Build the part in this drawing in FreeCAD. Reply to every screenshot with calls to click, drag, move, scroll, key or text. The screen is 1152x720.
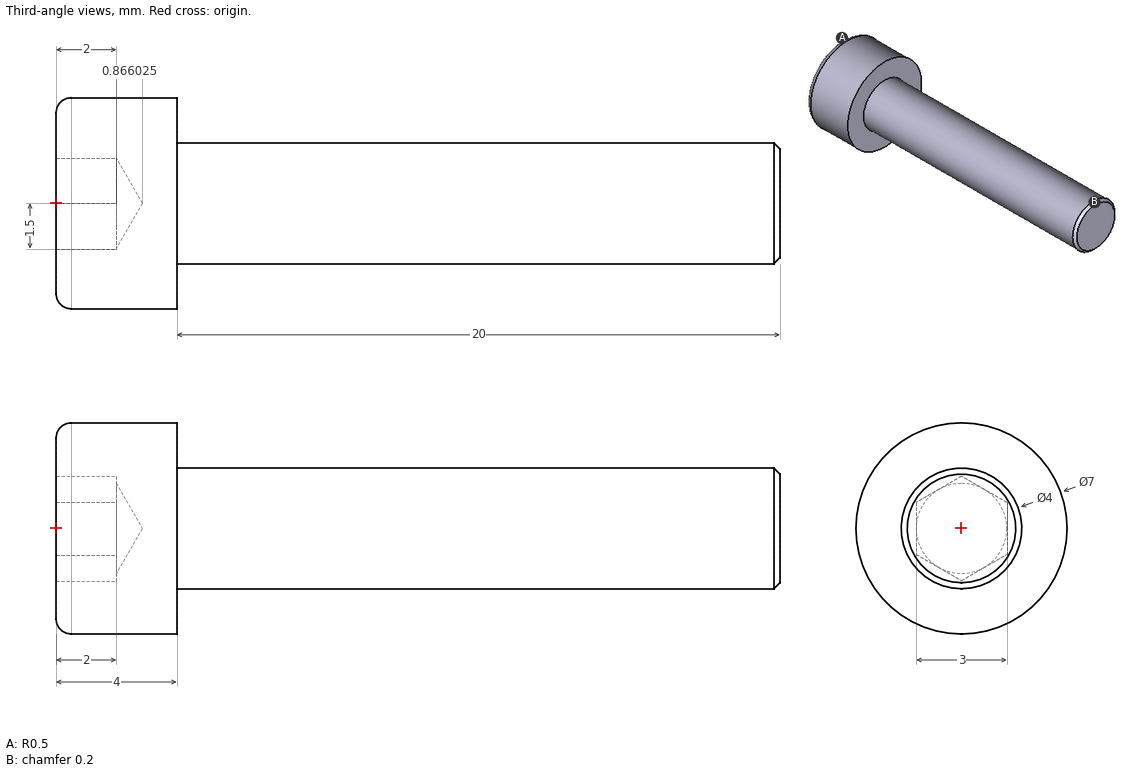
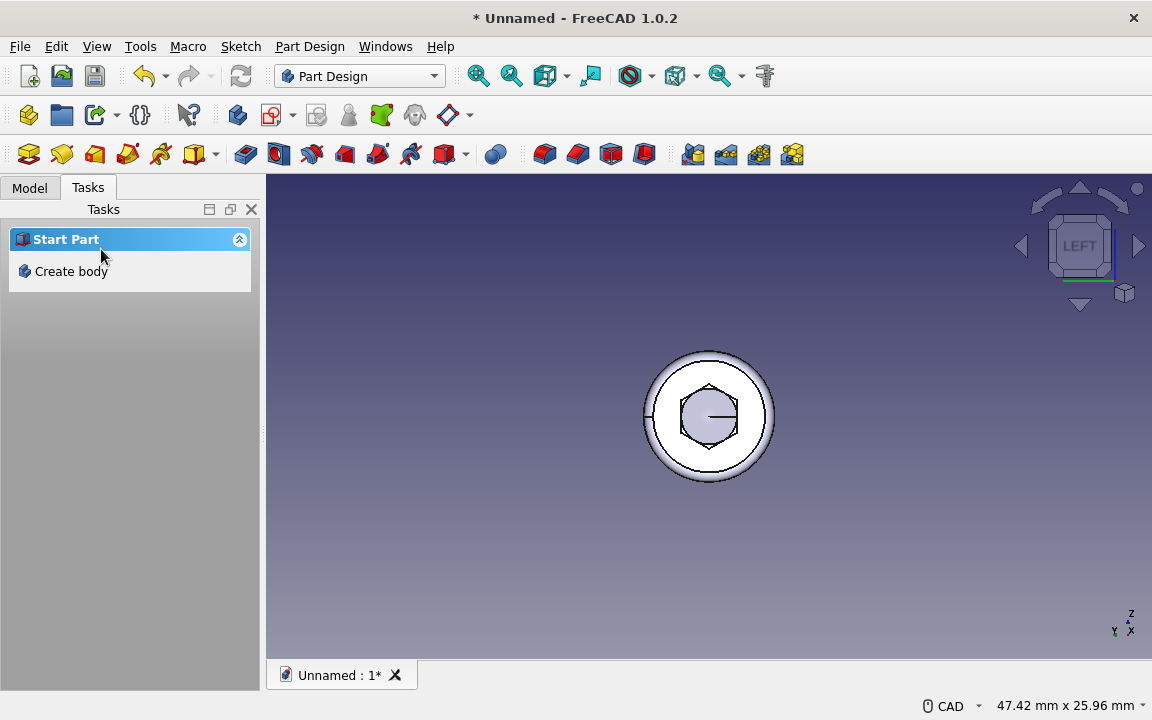
click(479, 76)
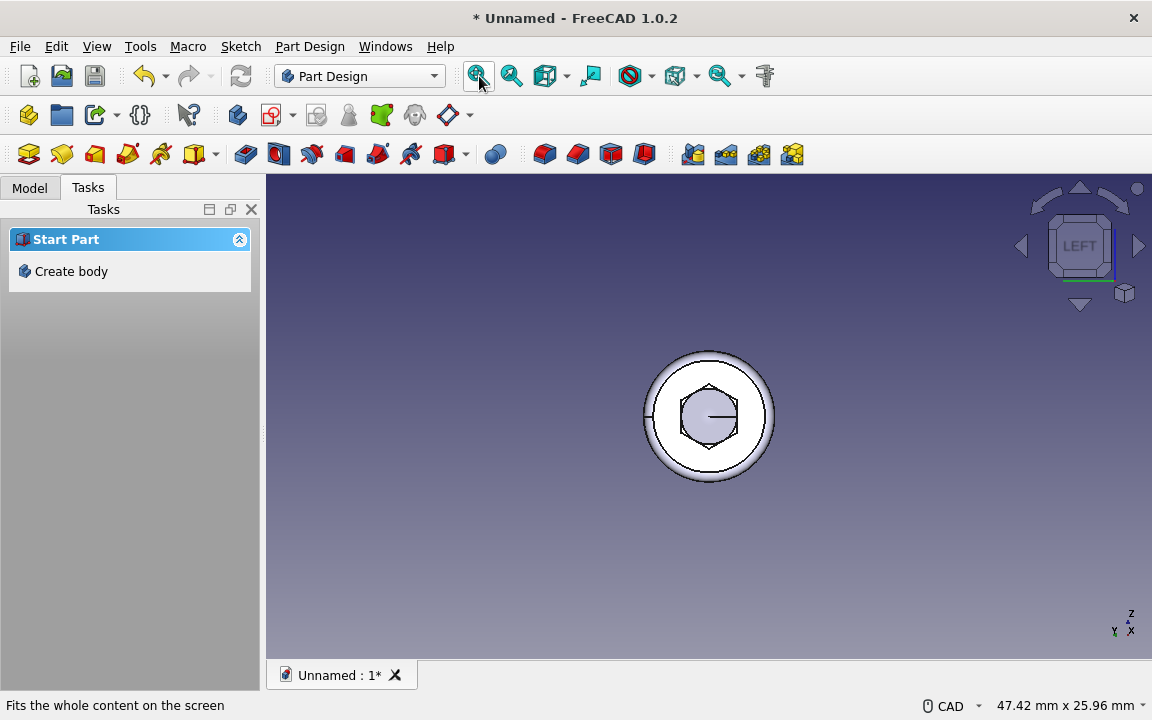
key(0)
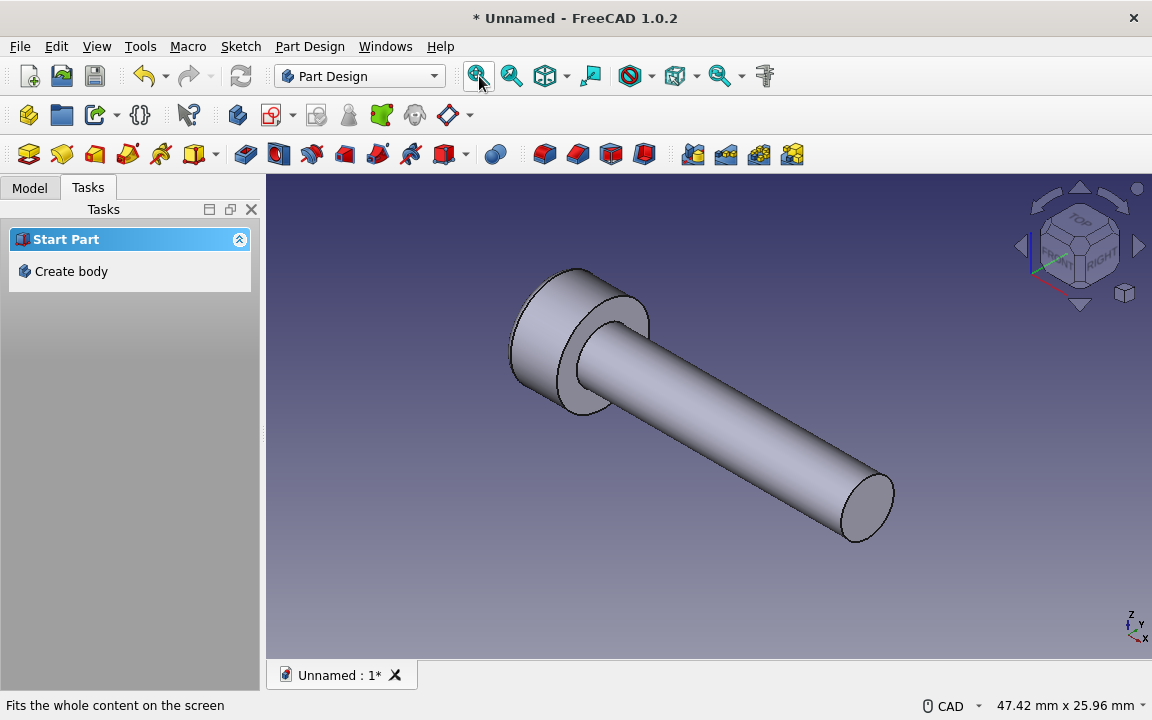
click(841, 522)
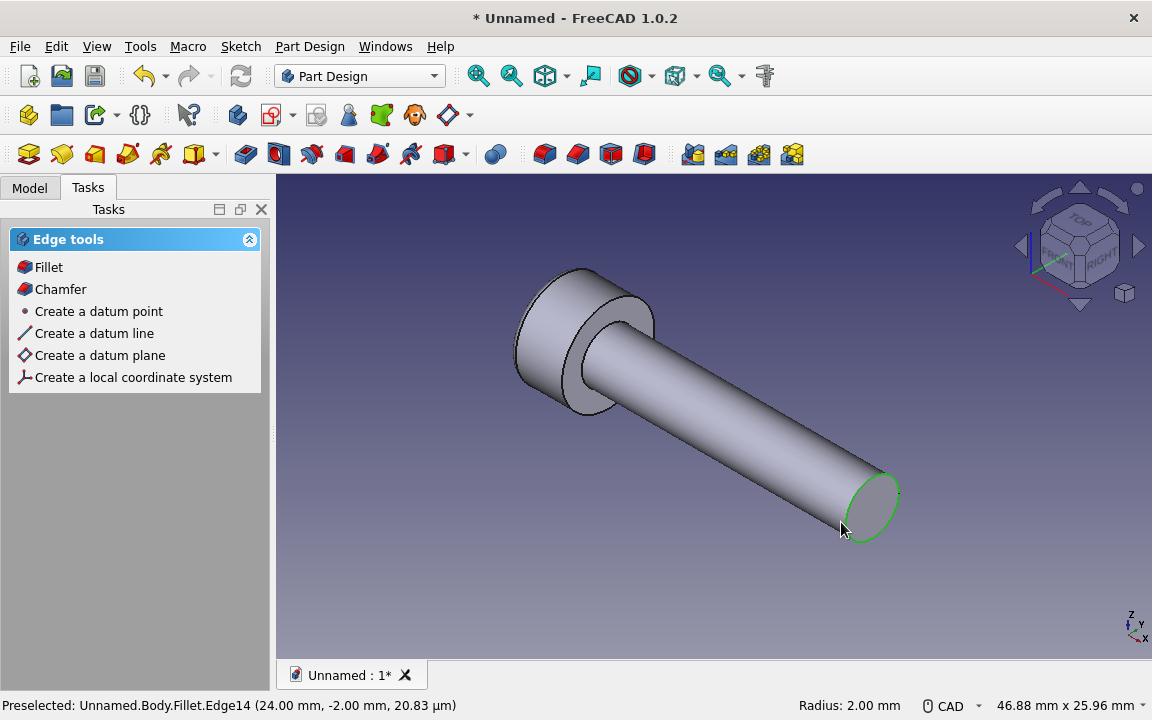
click(578, 154)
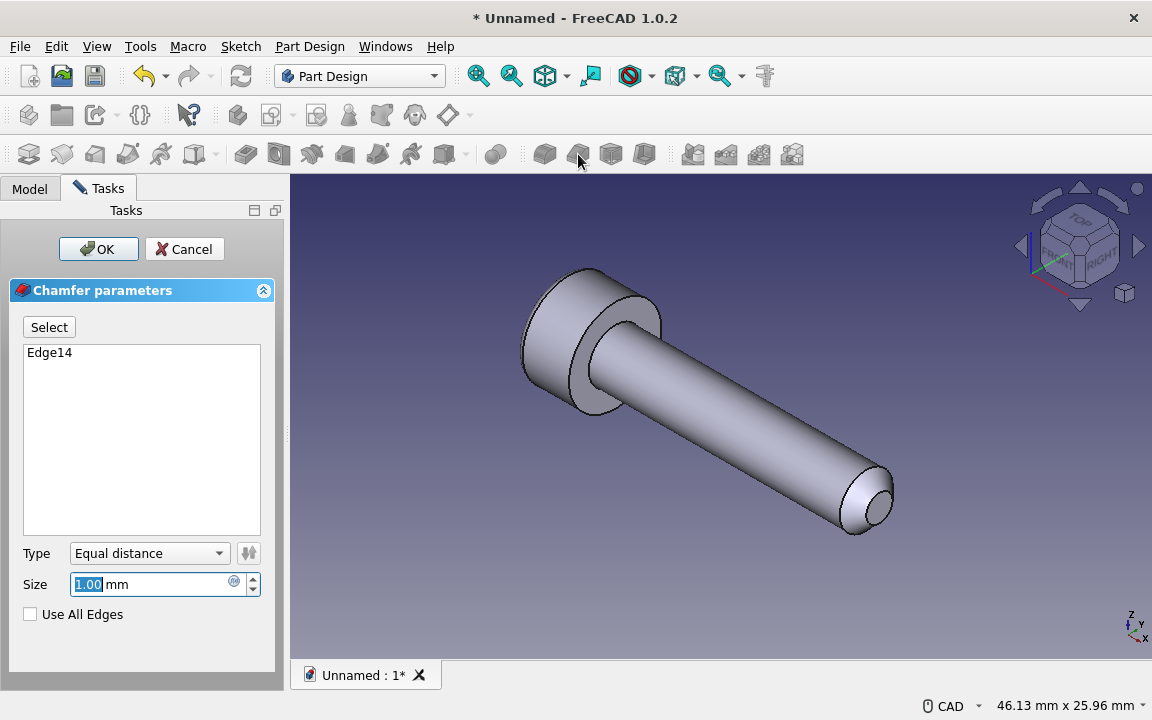
text(0.2)
key(Tab)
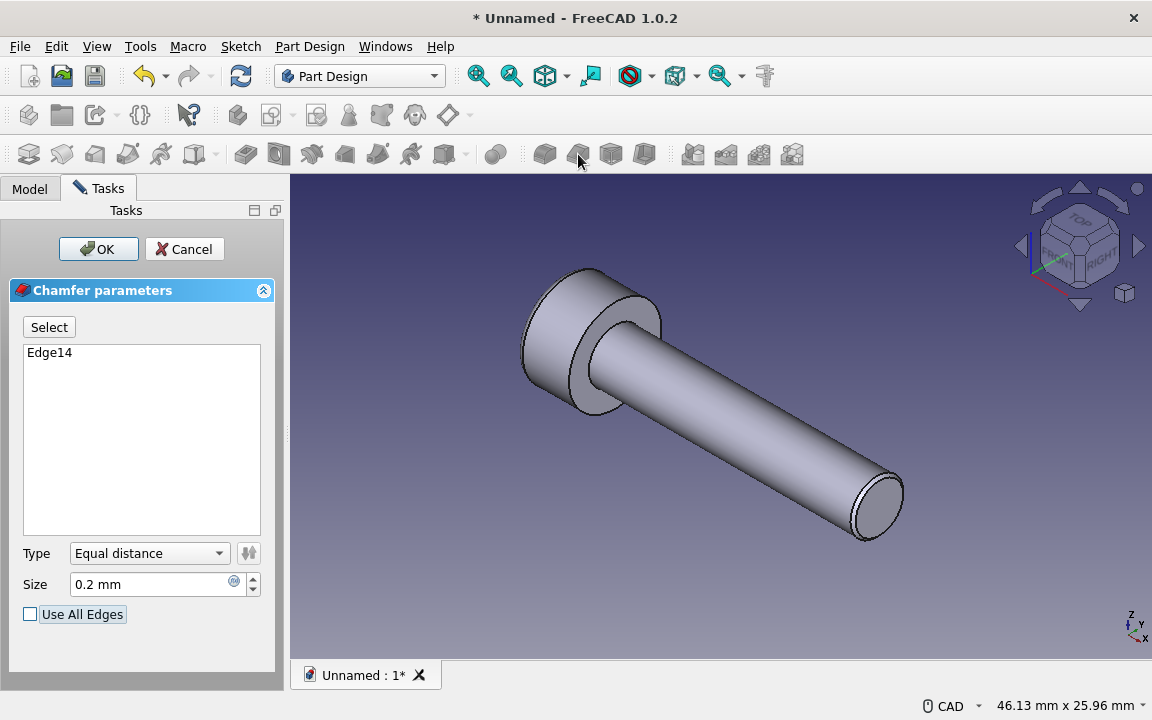
click(99, 249)